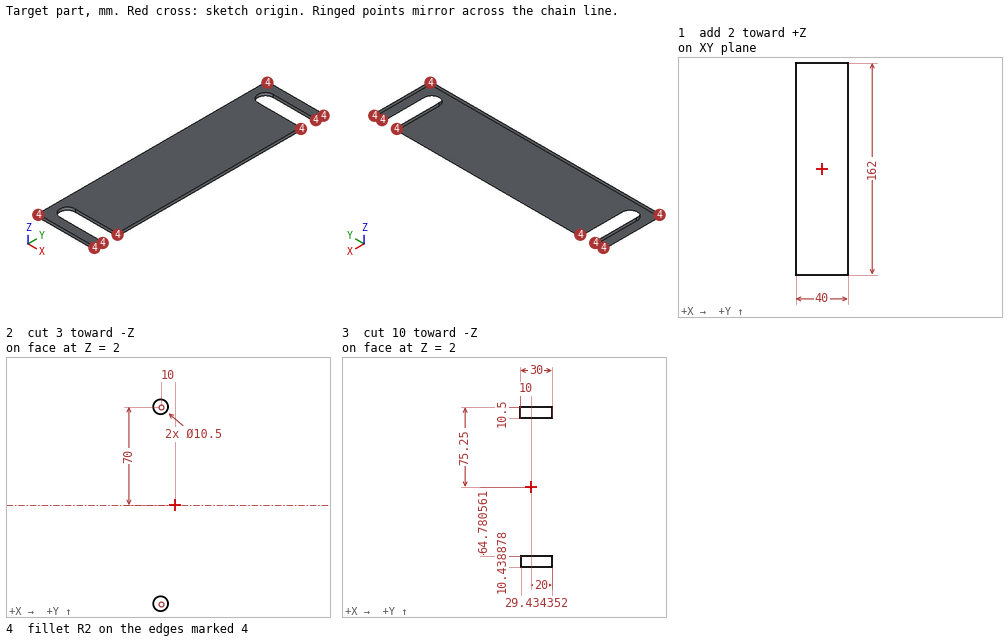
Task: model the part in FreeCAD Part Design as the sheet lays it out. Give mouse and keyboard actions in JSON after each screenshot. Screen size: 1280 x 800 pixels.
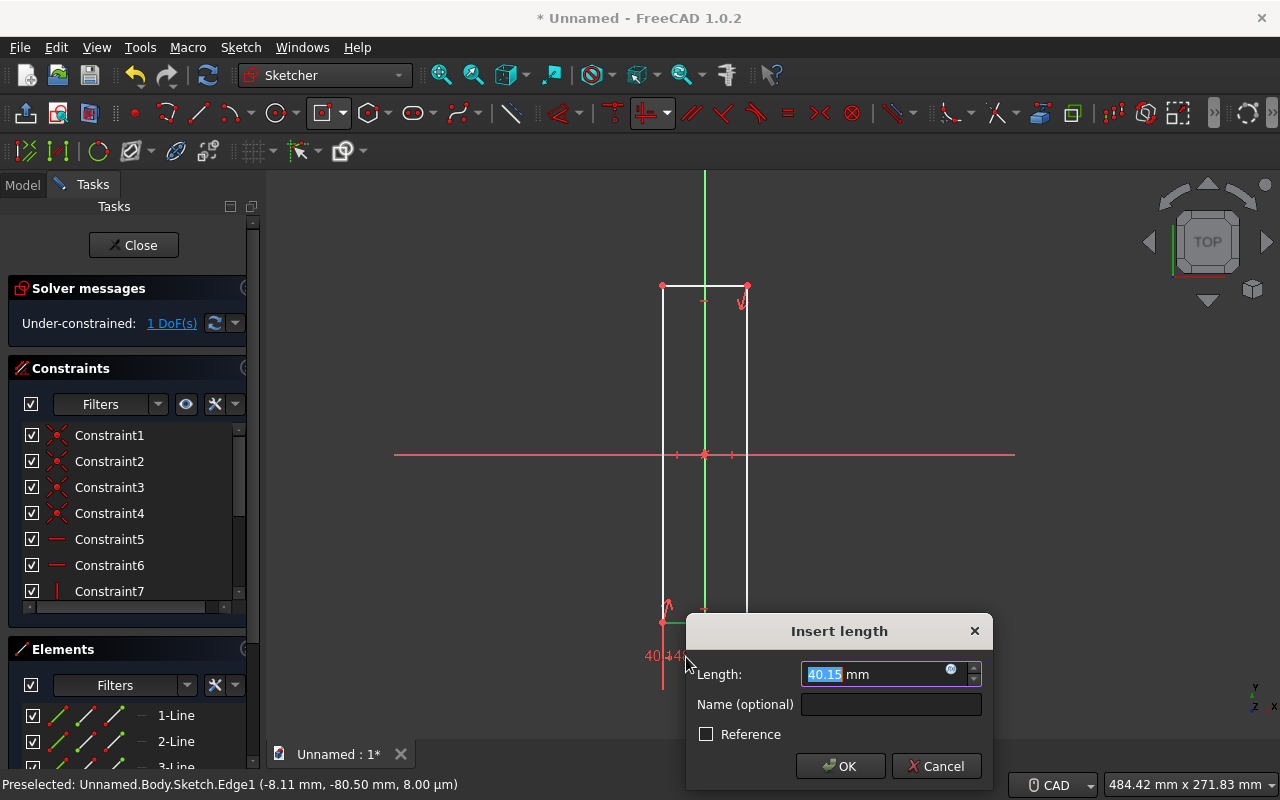
{"action": "type", "text": "40"}
{"action": "key", "text": "Return"}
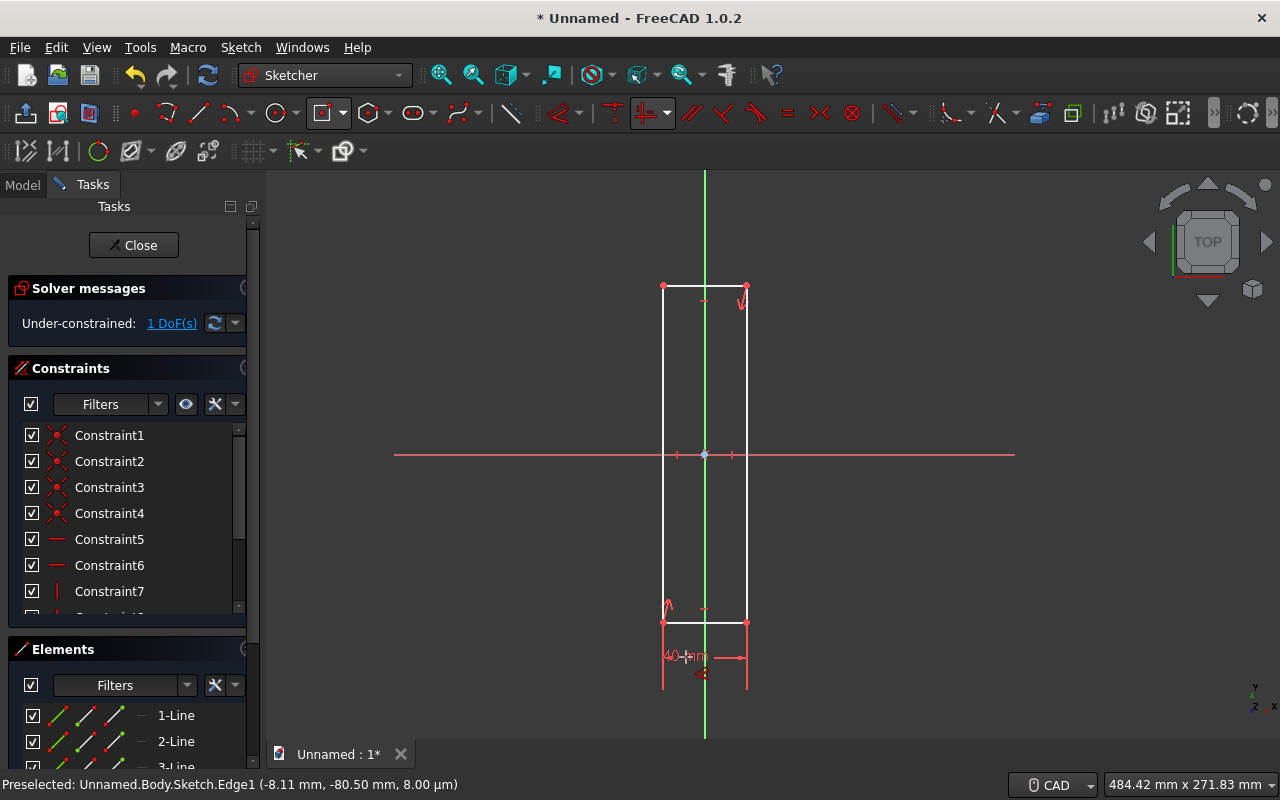
{"action": "left_click", "coordinate": [747, 522]}
{"action": "left_click", "coordinate": [781, 377]}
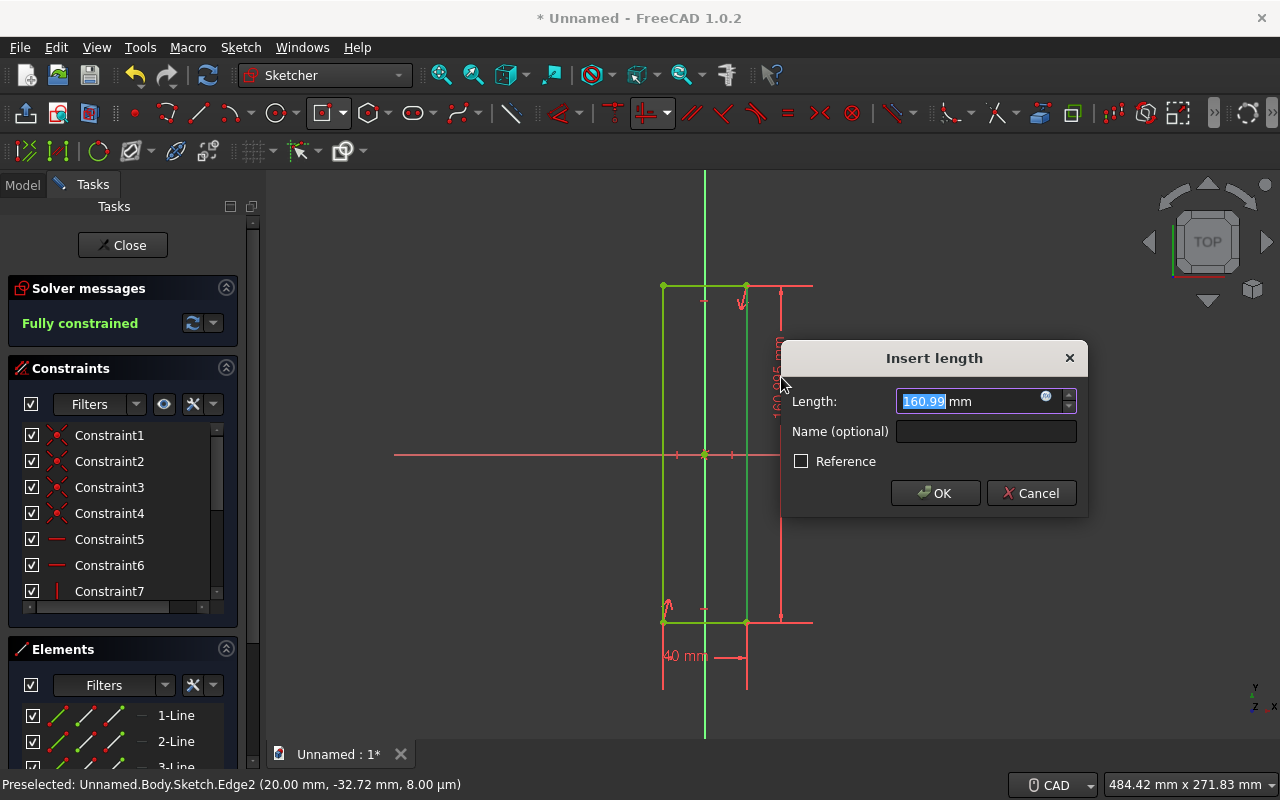
{"action": "type", "text": "162"}
{"action": "key", "text": "Return"}
{"action": "key", "text": "Escape"}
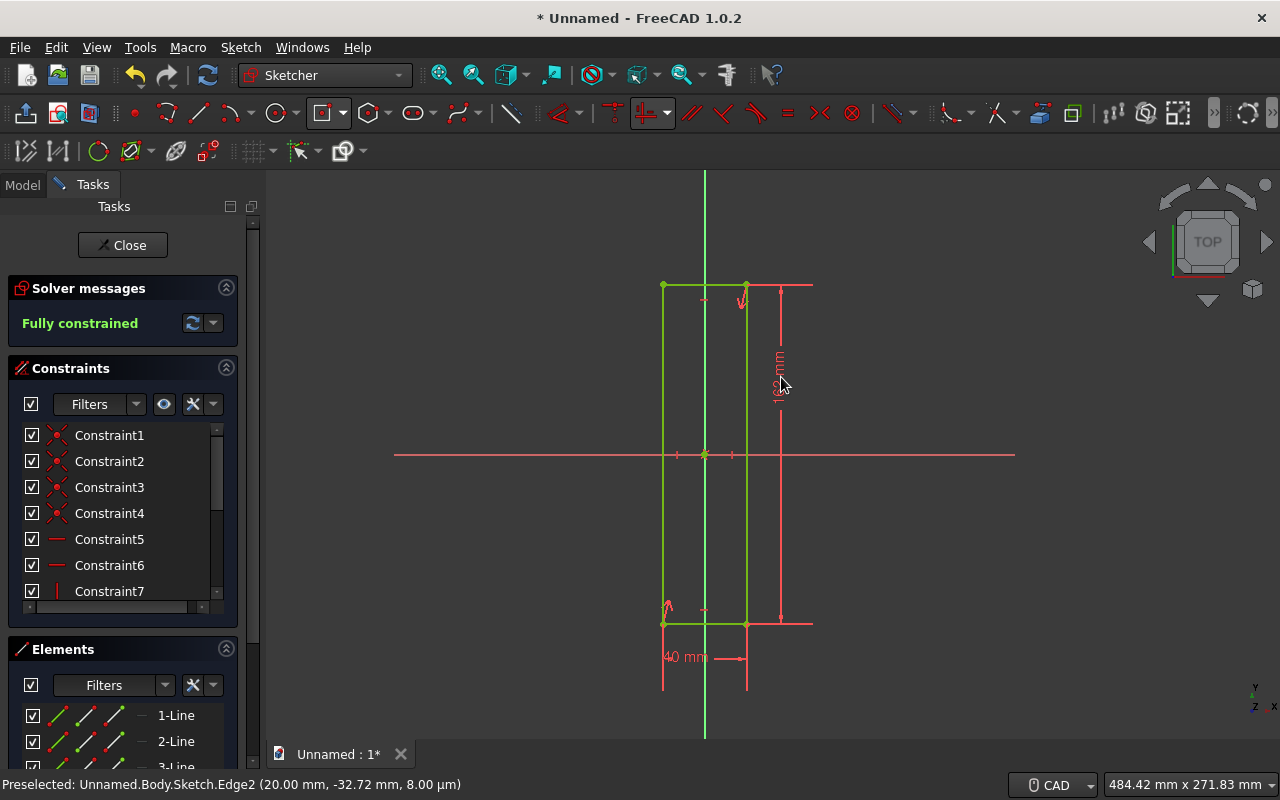
{"action": "left_click", "coordinate": [123, 245]}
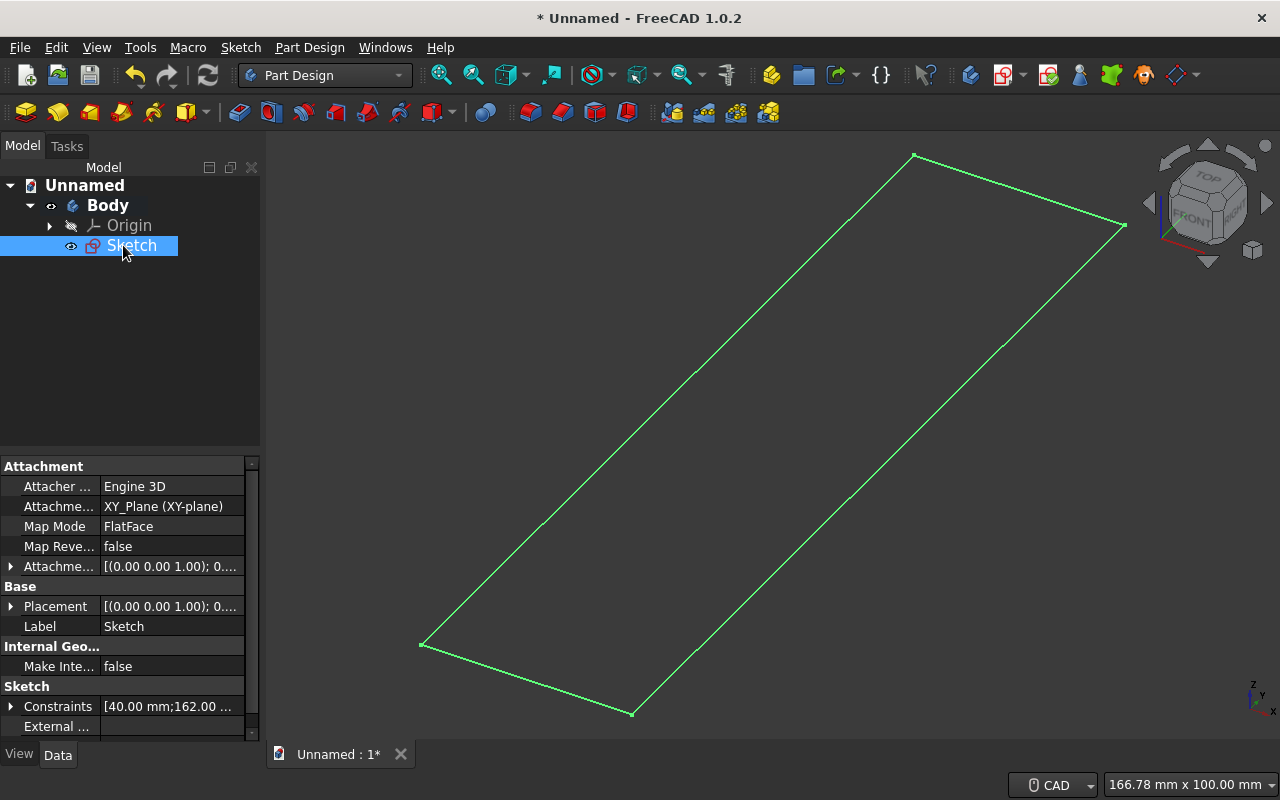
{"action": "left_click", "coordinate": [26, 112]}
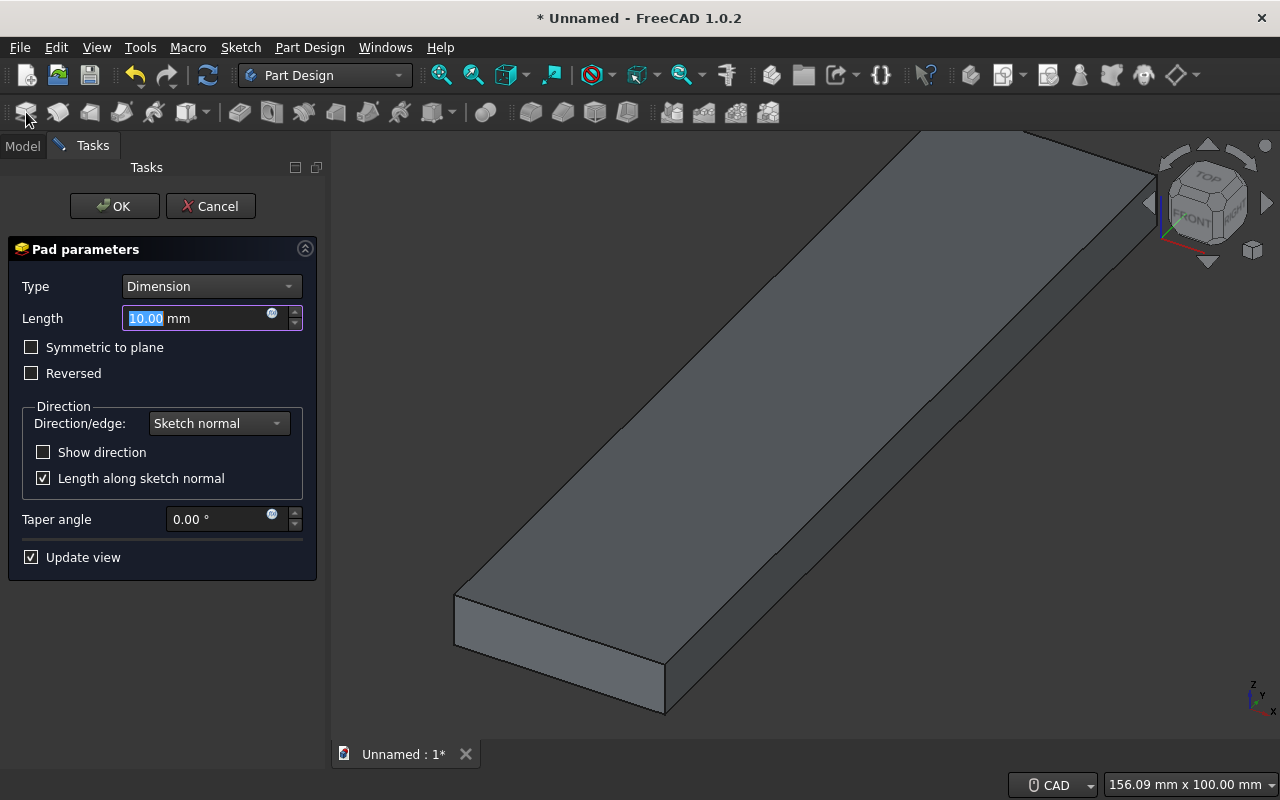
{"action": "type", "text": "2"}
{"action": "key", "text": "Tab"}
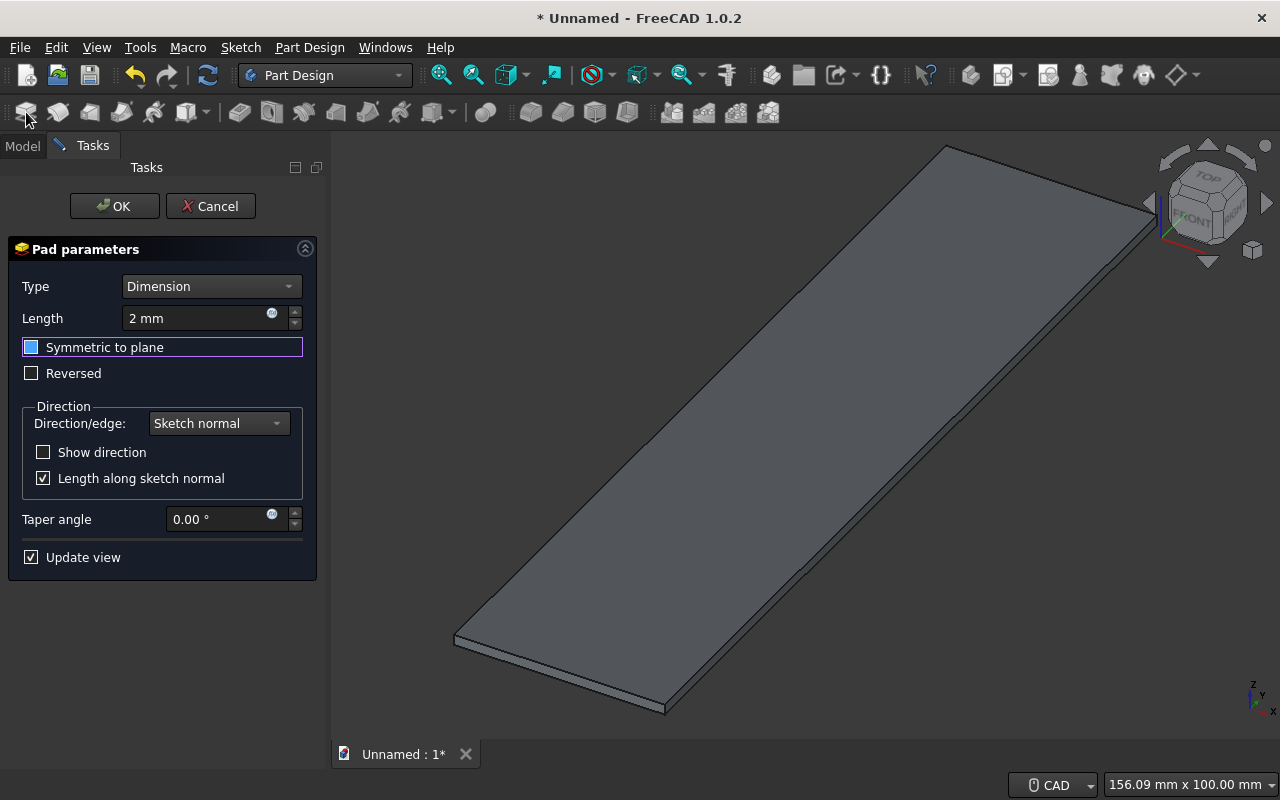
{"action": "left_click", "coordinate": [115, 206]}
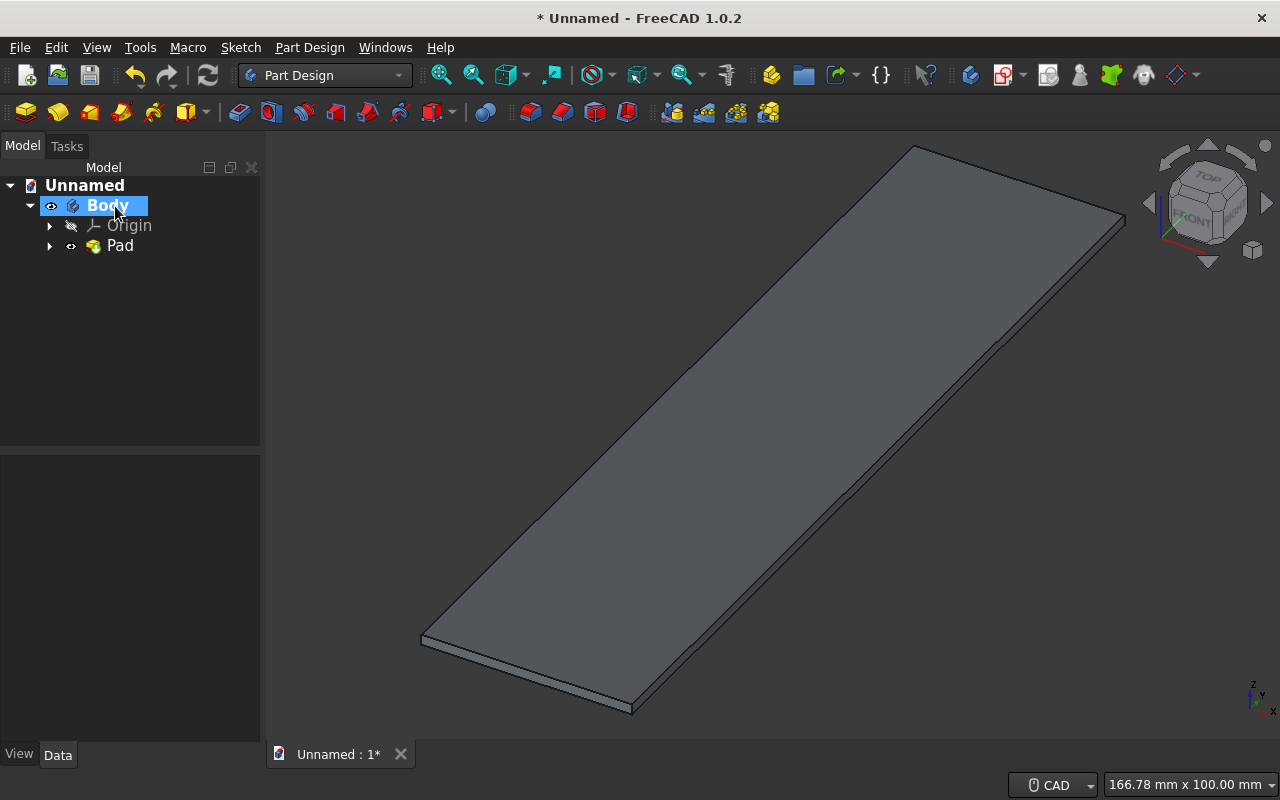
{"action": "left_click", "coordinate": [914, 284]}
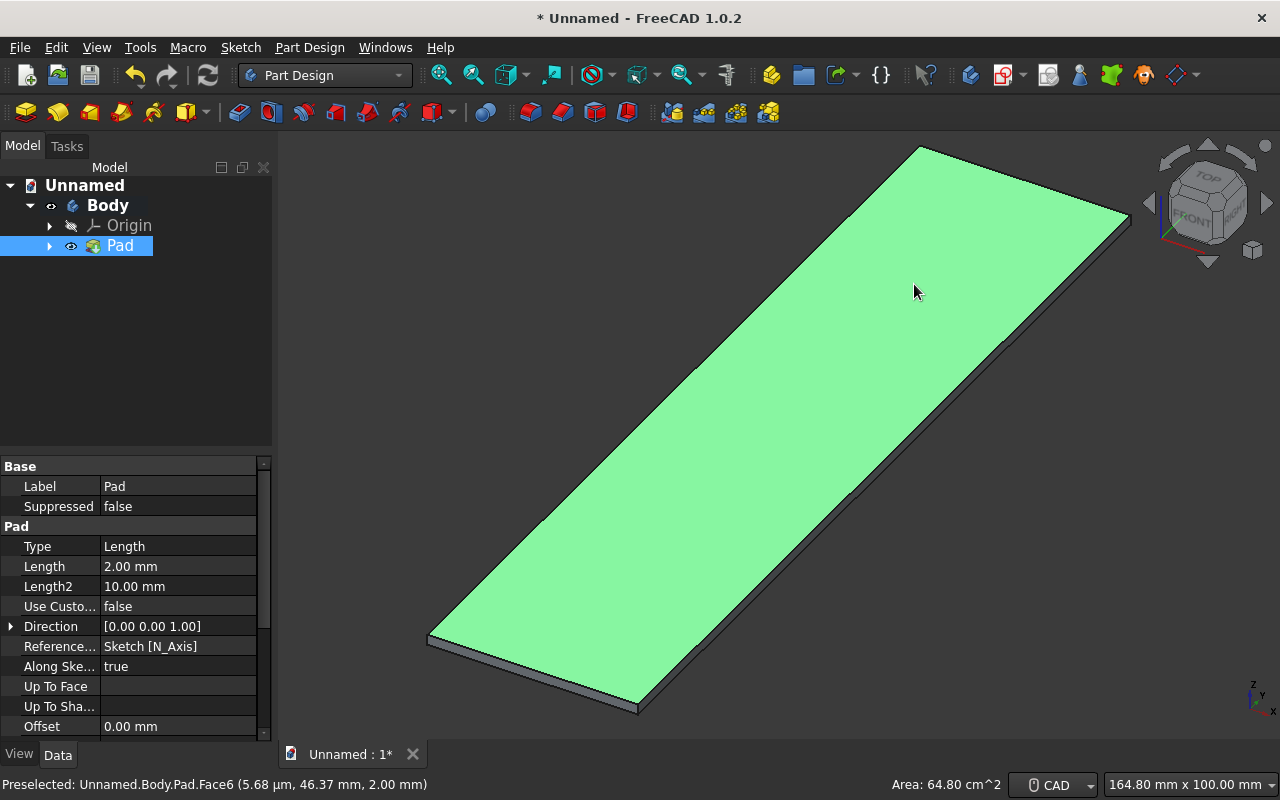
{"action": "left_click", "coordinate": [1004, 76]}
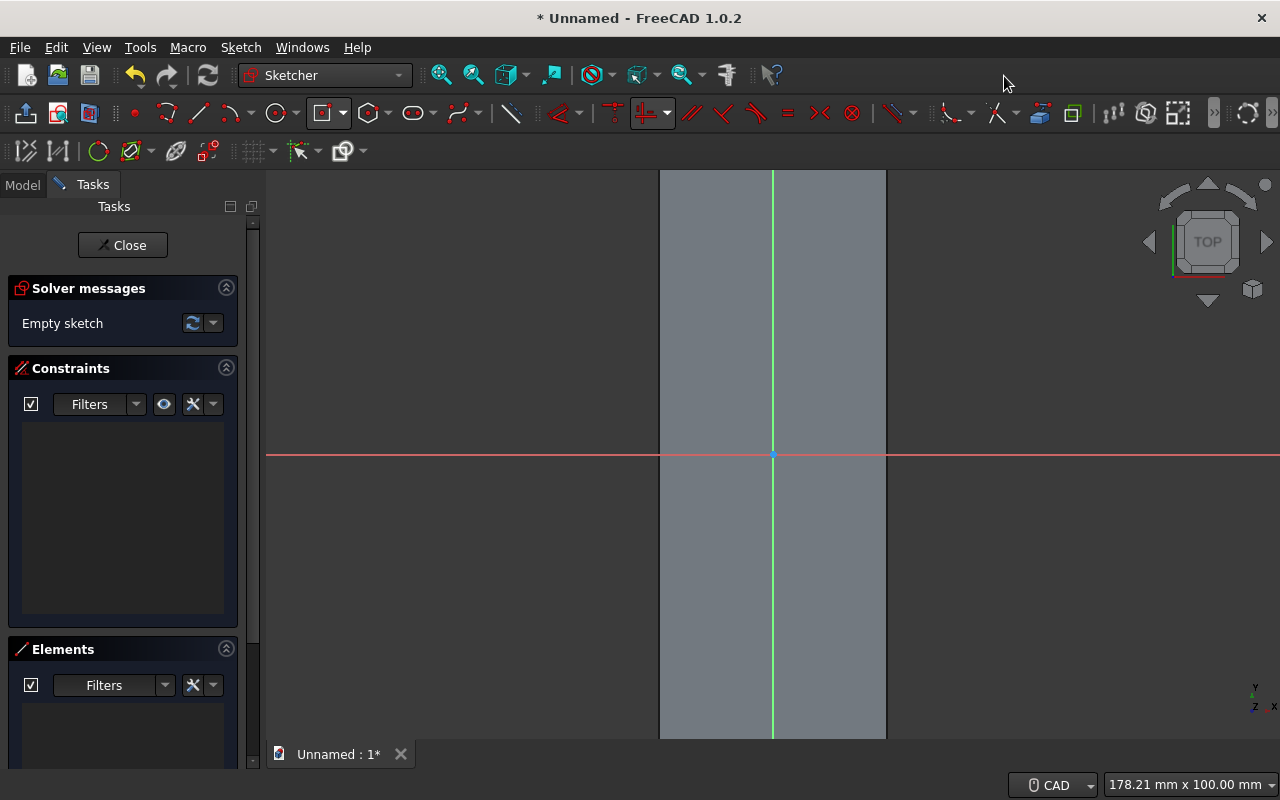
{"action": "scroll", "coordinate": [684, 454], "scroll_direction": "down", "scroll_amount": 4}